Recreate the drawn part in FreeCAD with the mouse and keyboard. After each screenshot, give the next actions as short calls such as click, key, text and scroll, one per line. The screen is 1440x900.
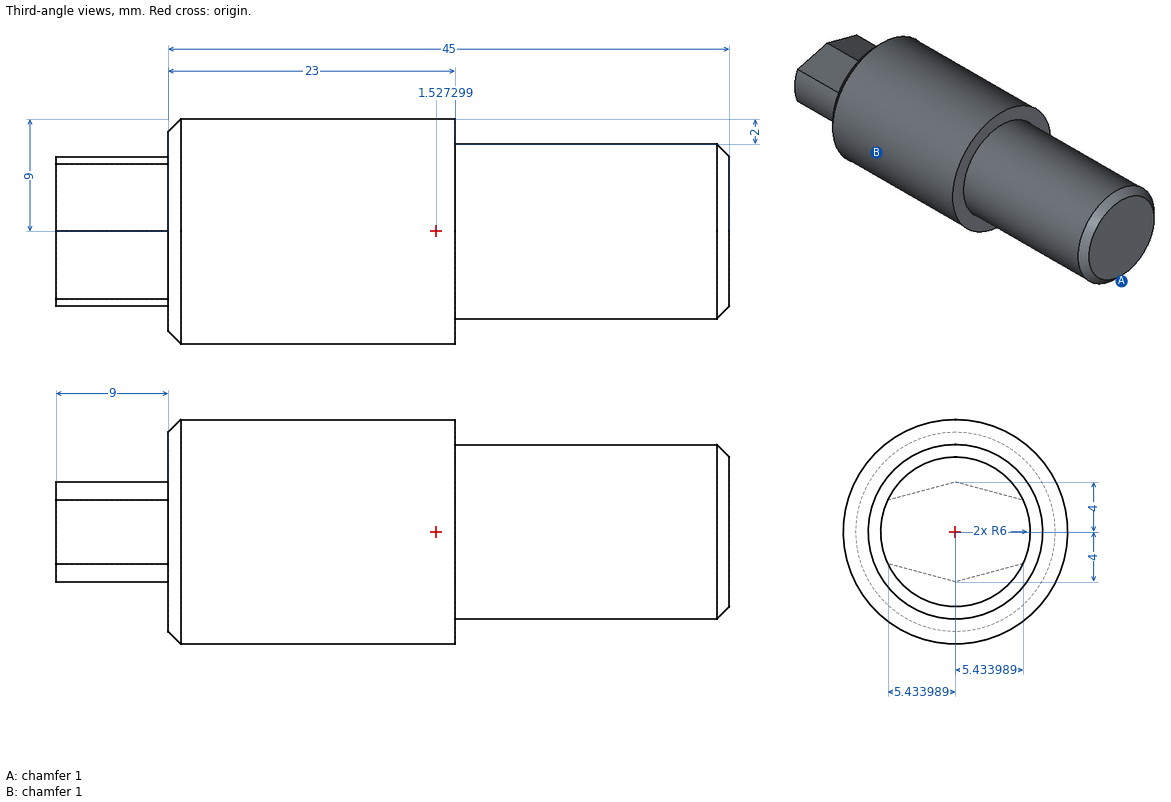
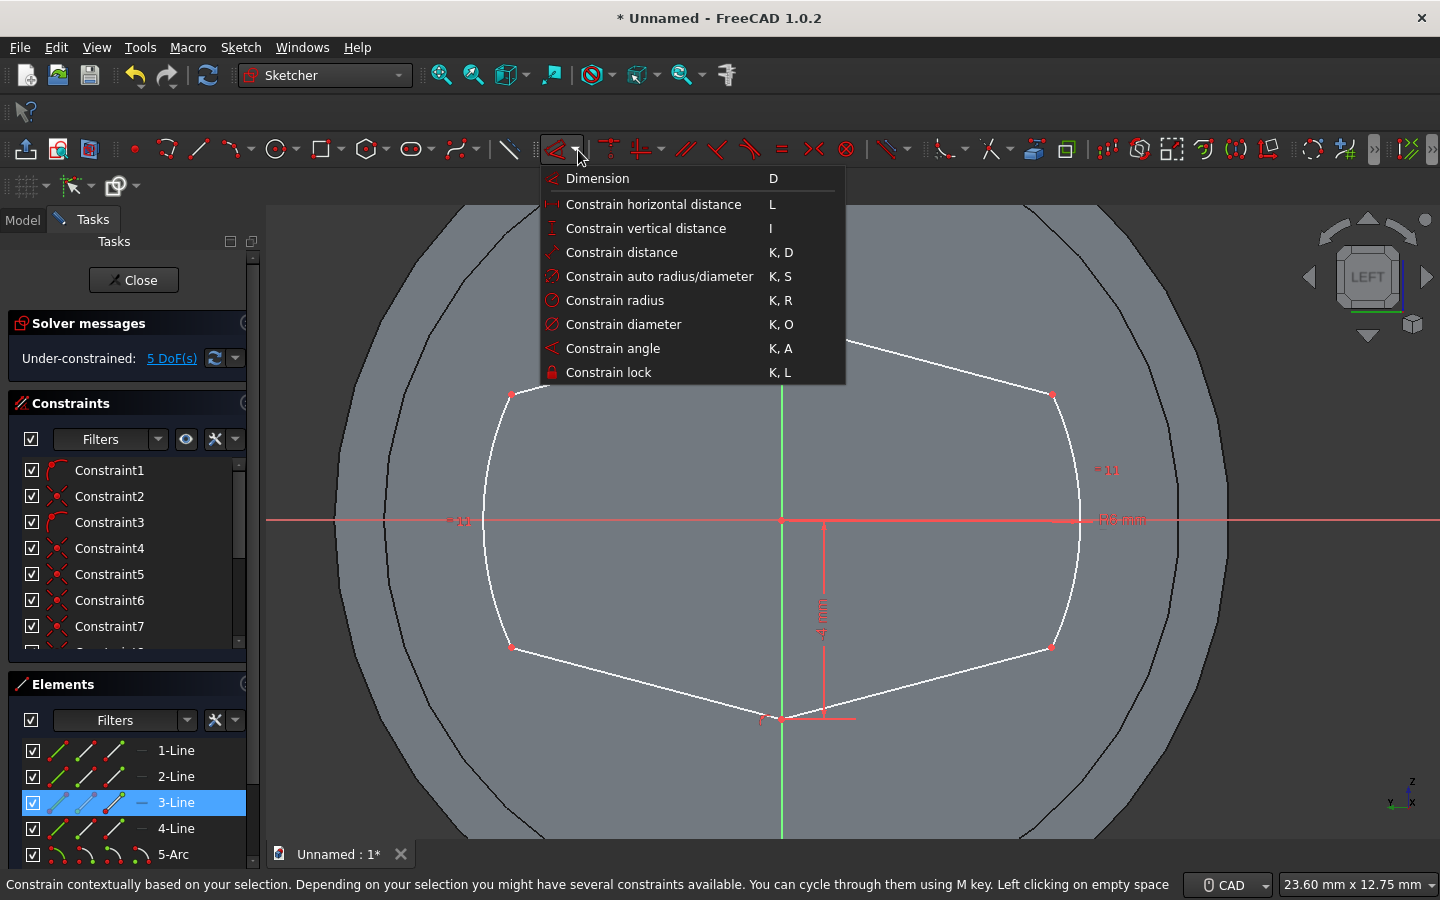
click(693, 228)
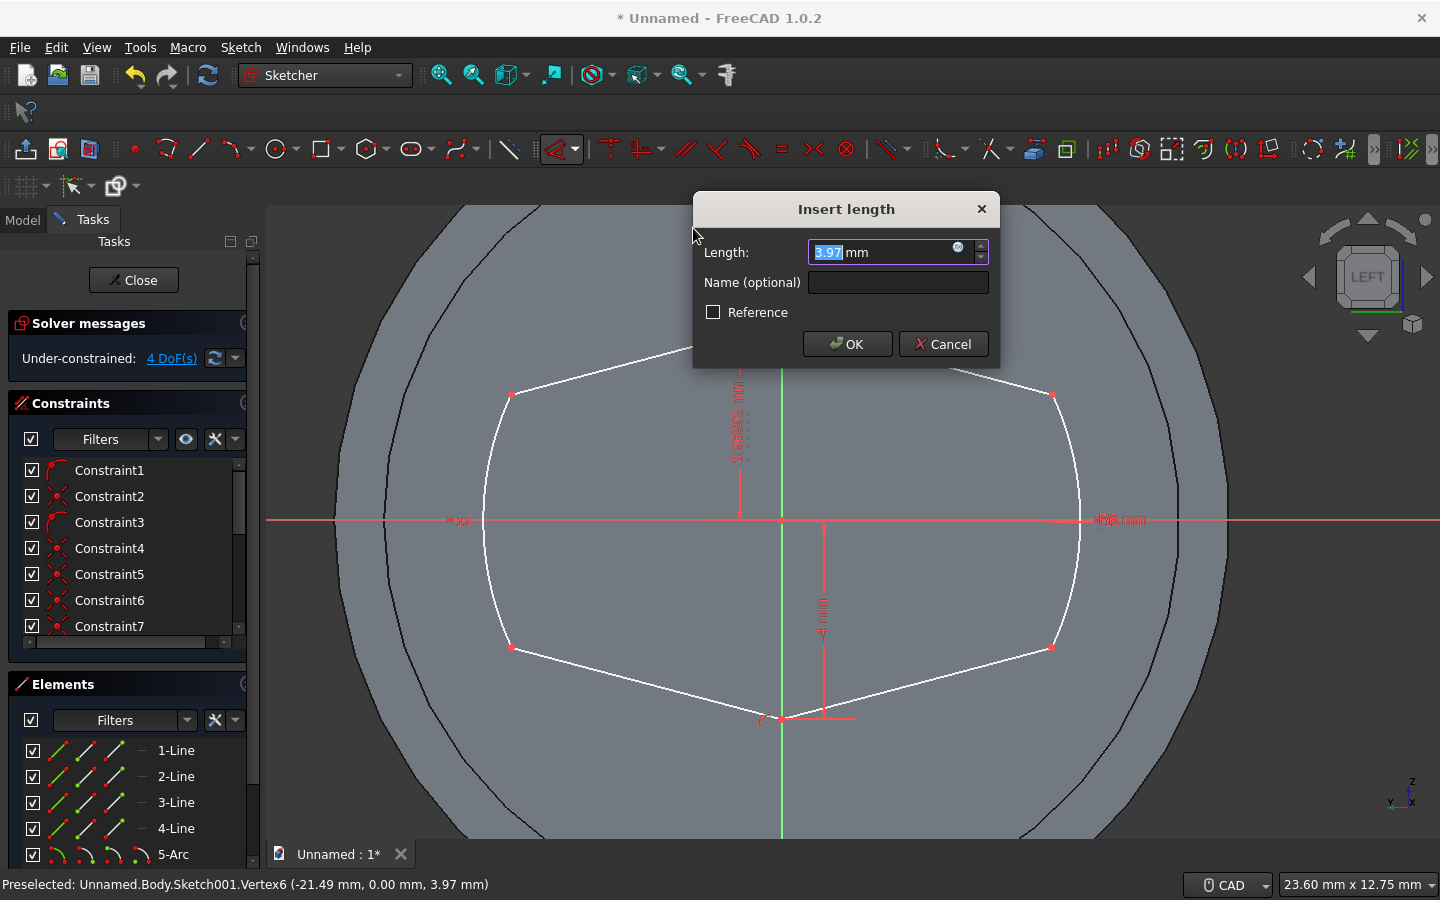
text(4)
key(Return)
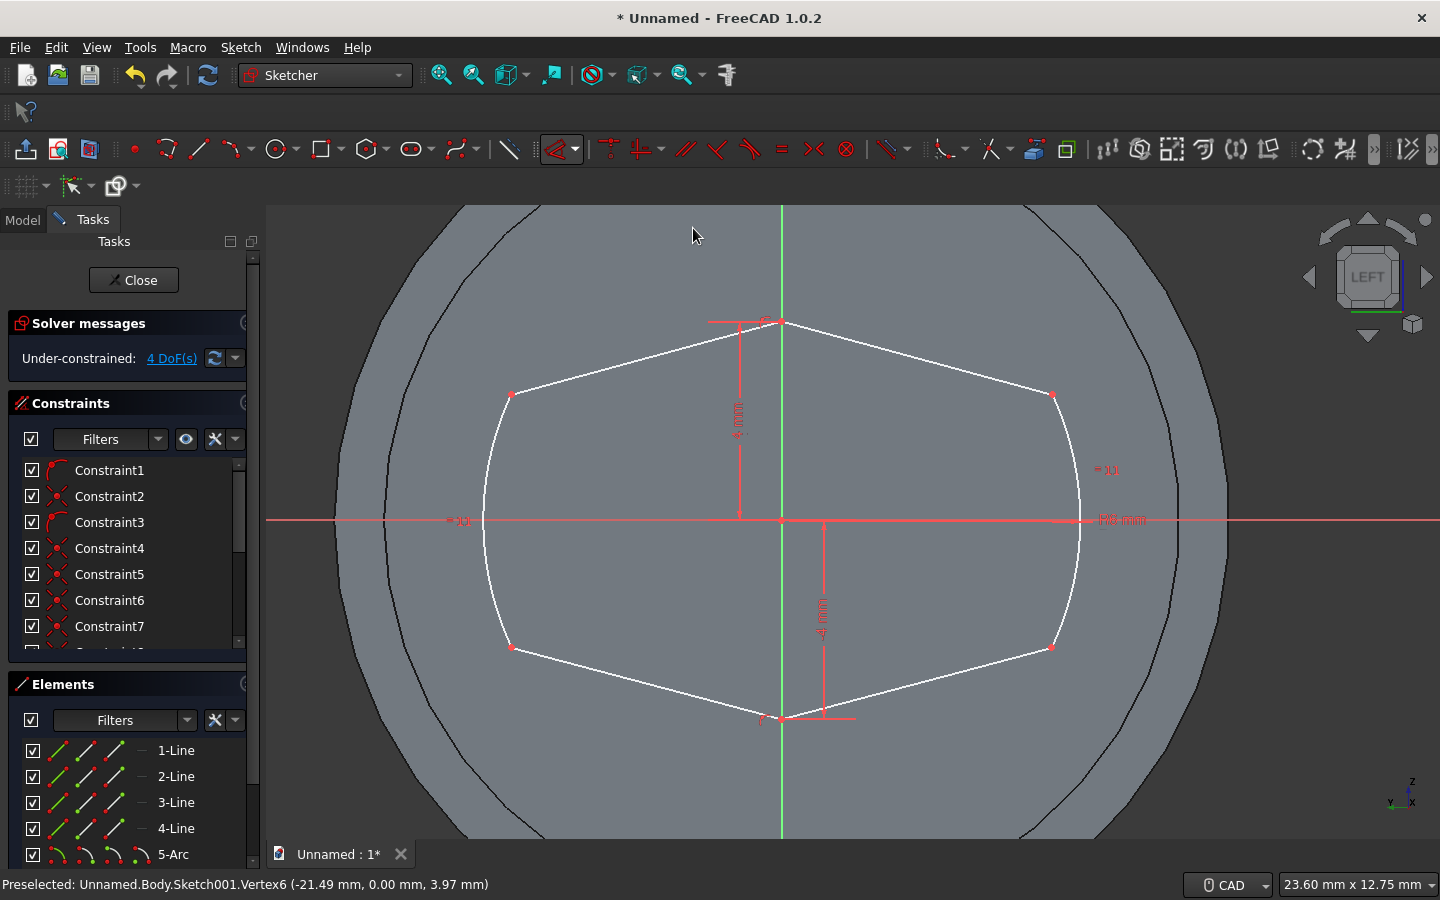
click(512, 648)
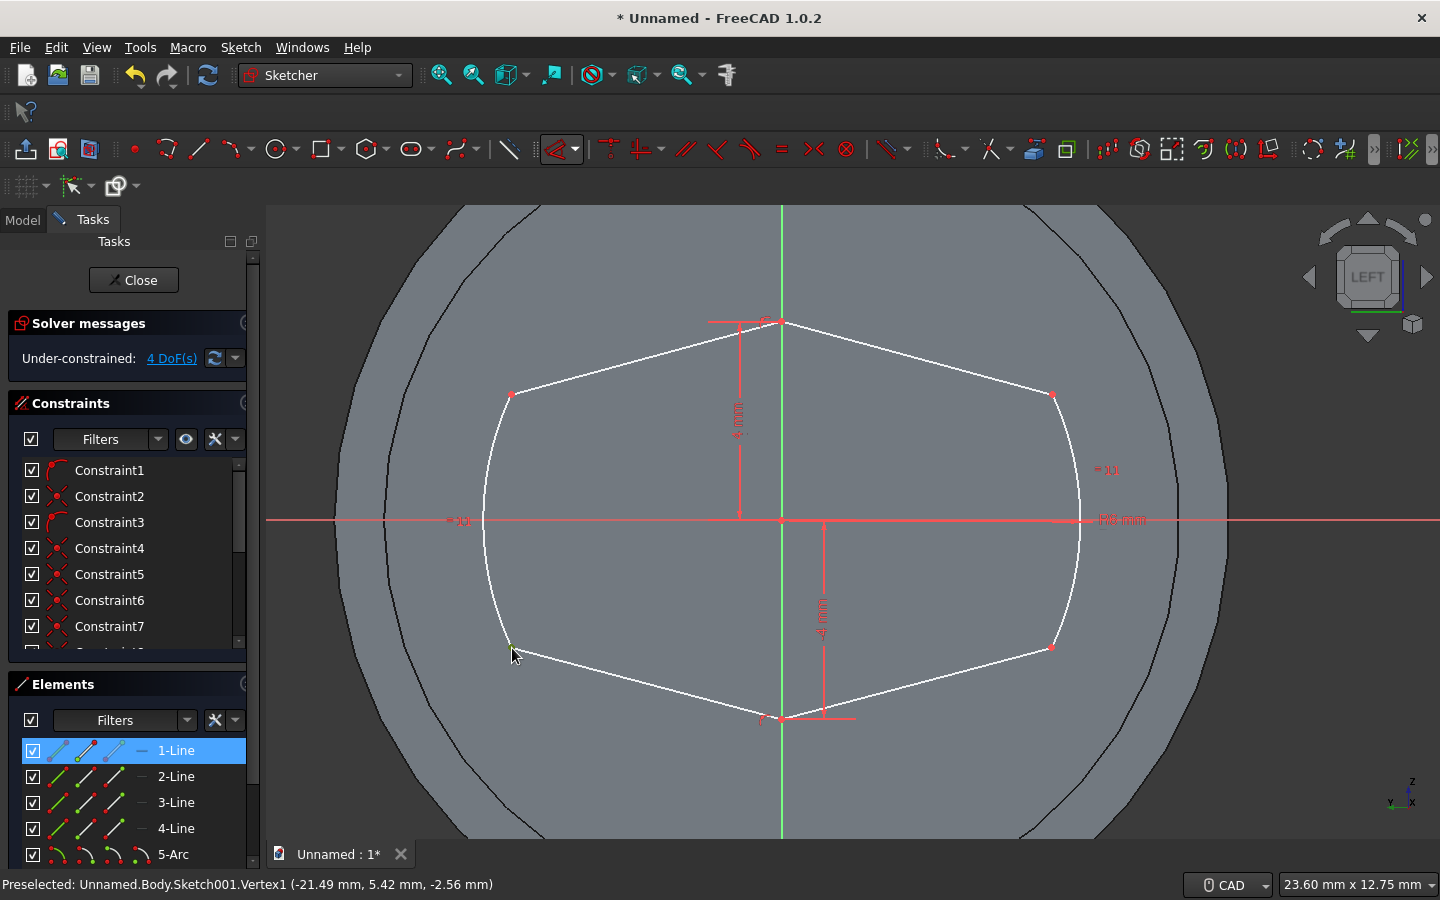
key(l)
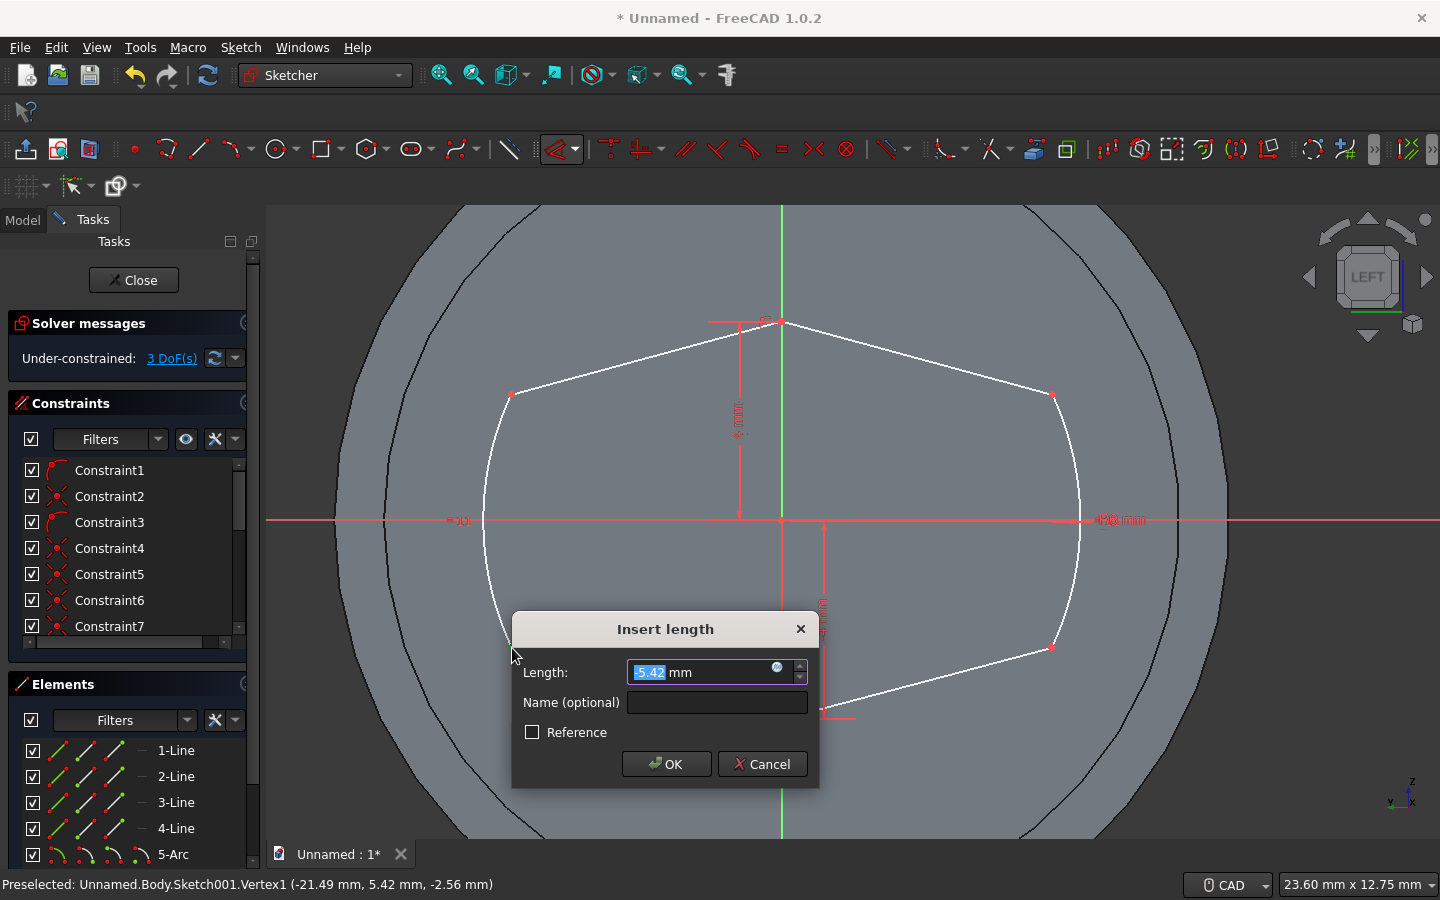
text(-5.433989)
key(Return)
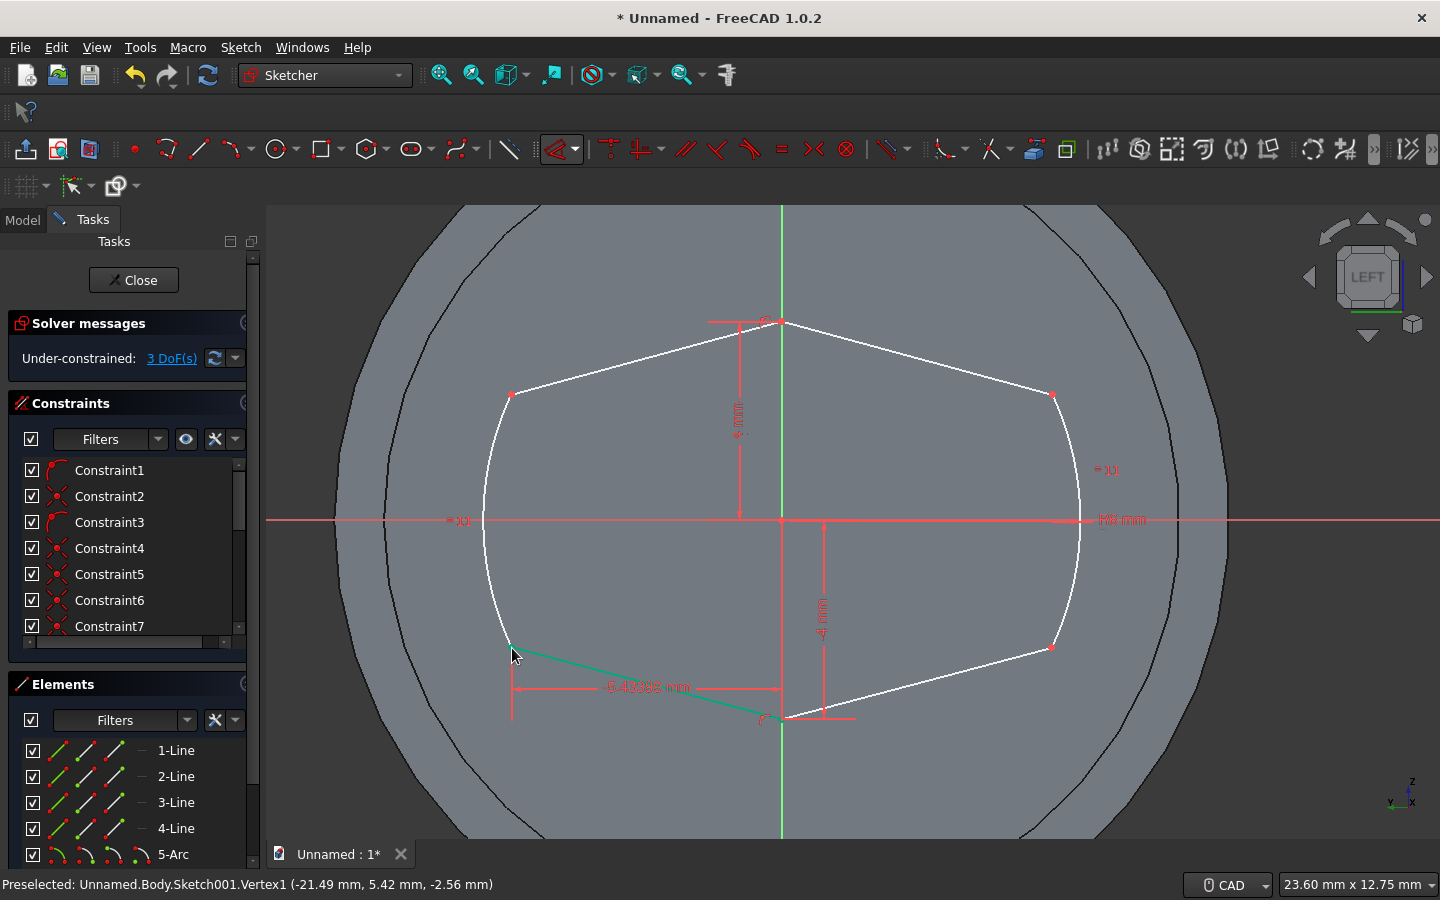
click(1052, 648)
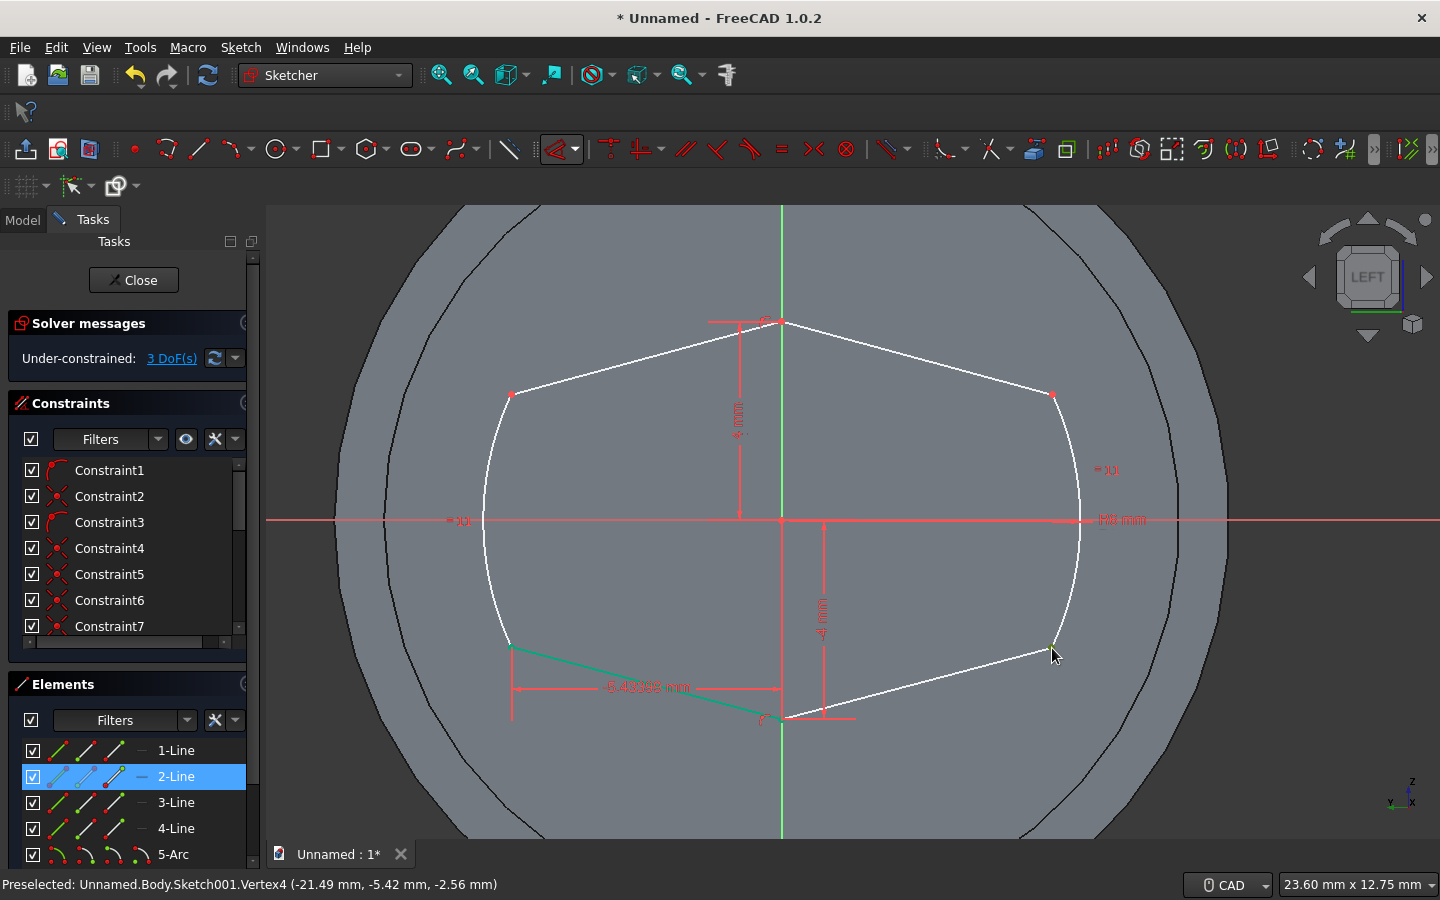
click(578, 150)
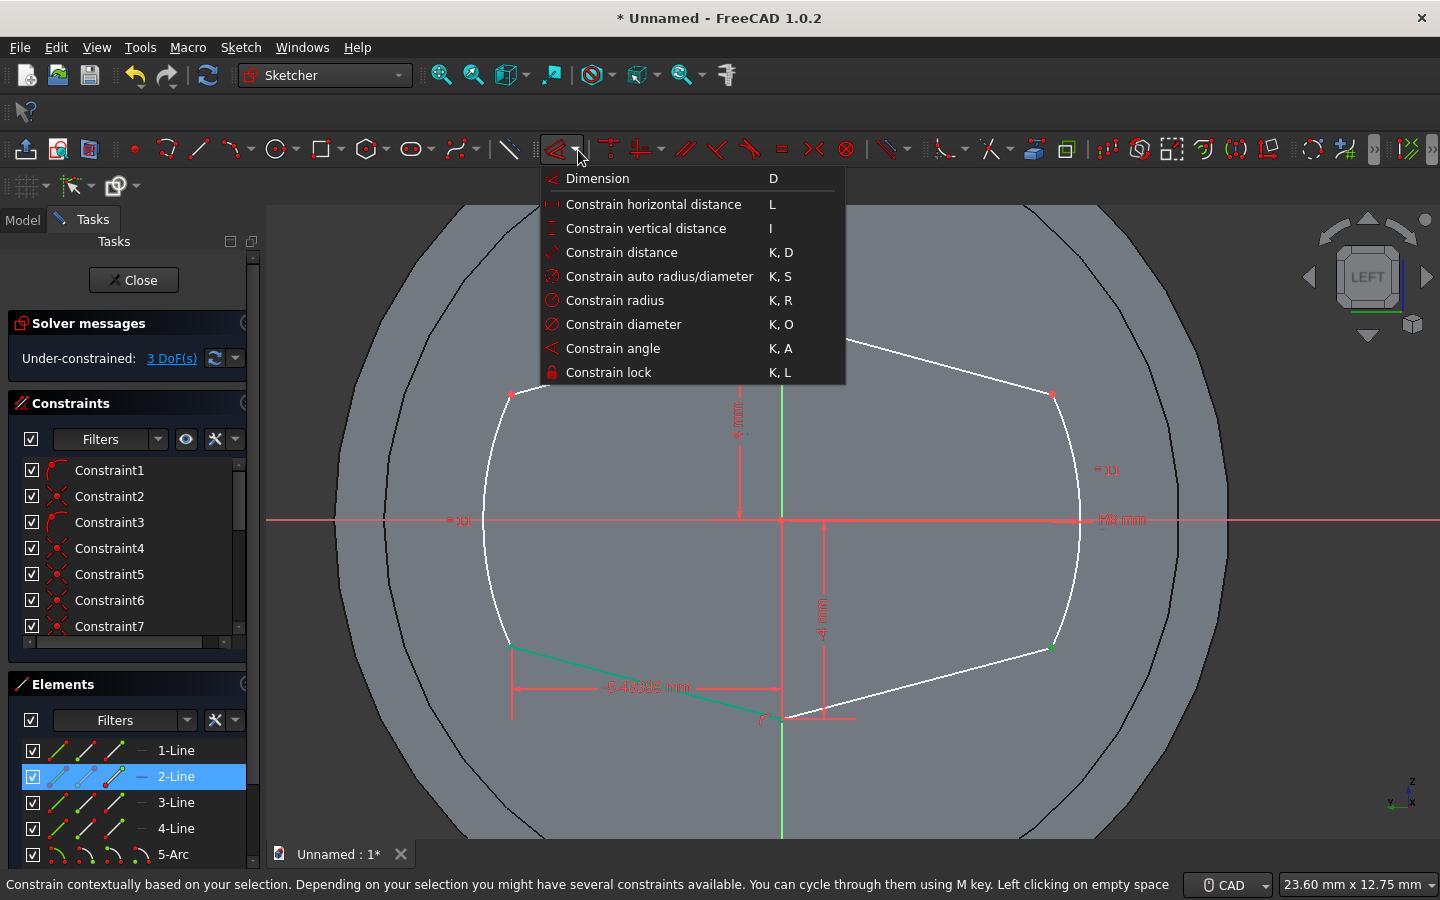
click(693, 204)